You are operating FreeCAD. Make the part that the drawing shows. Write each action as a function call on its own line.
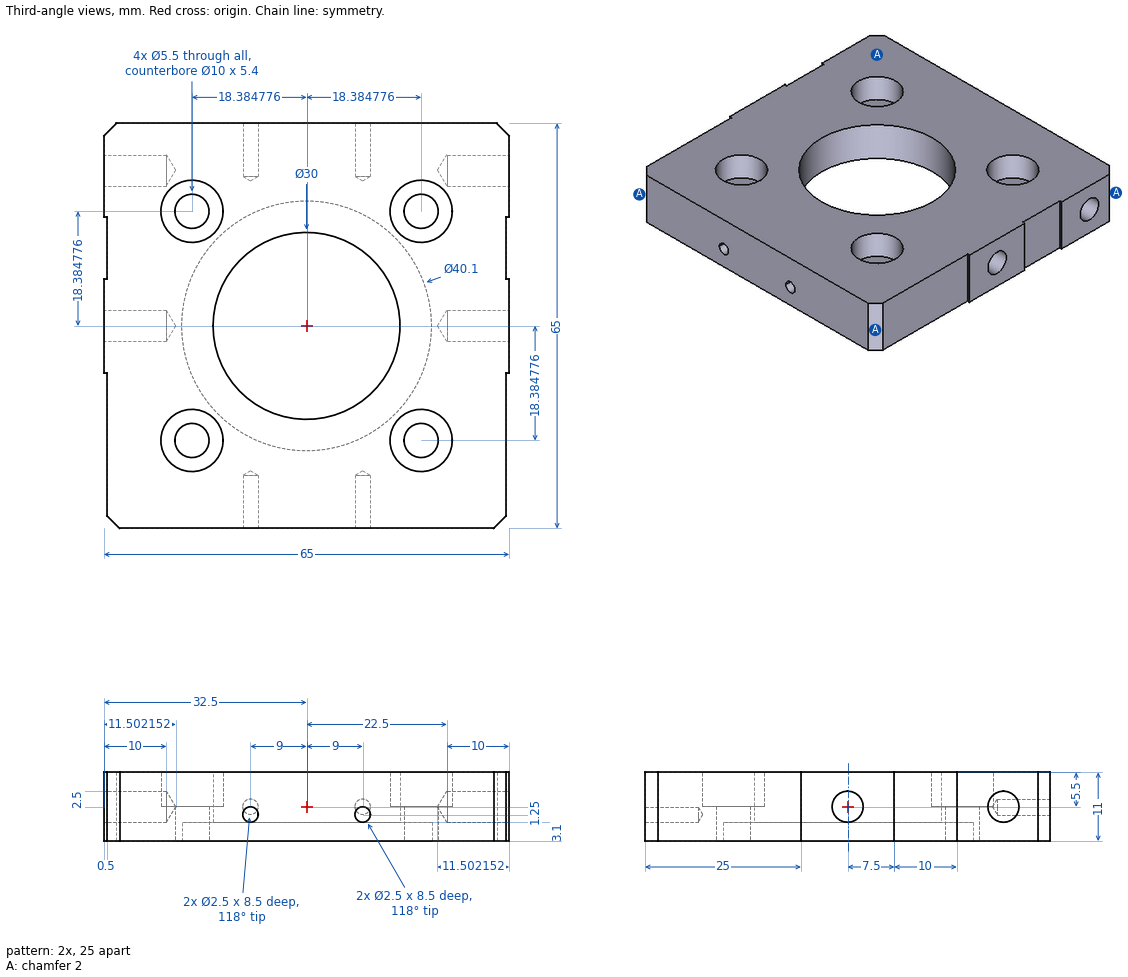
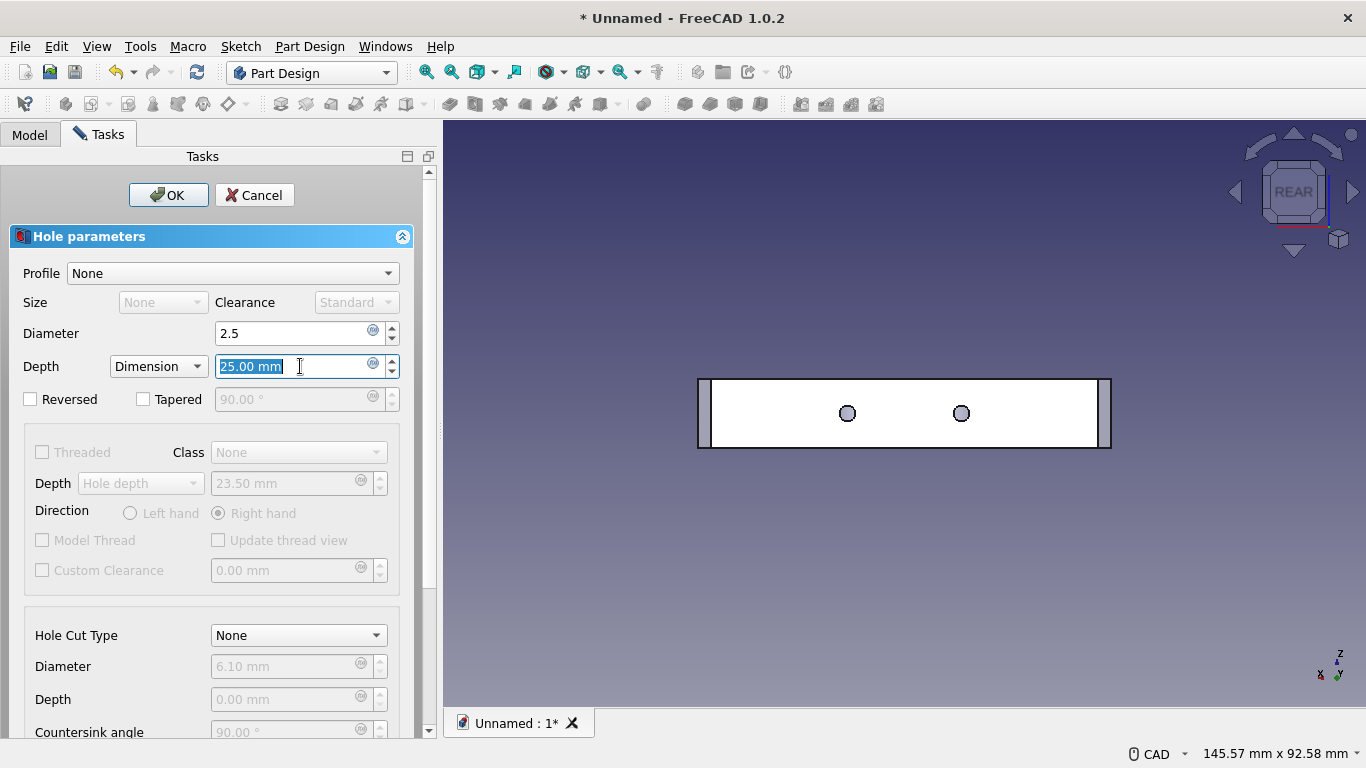
text(8.5)
key(Tab)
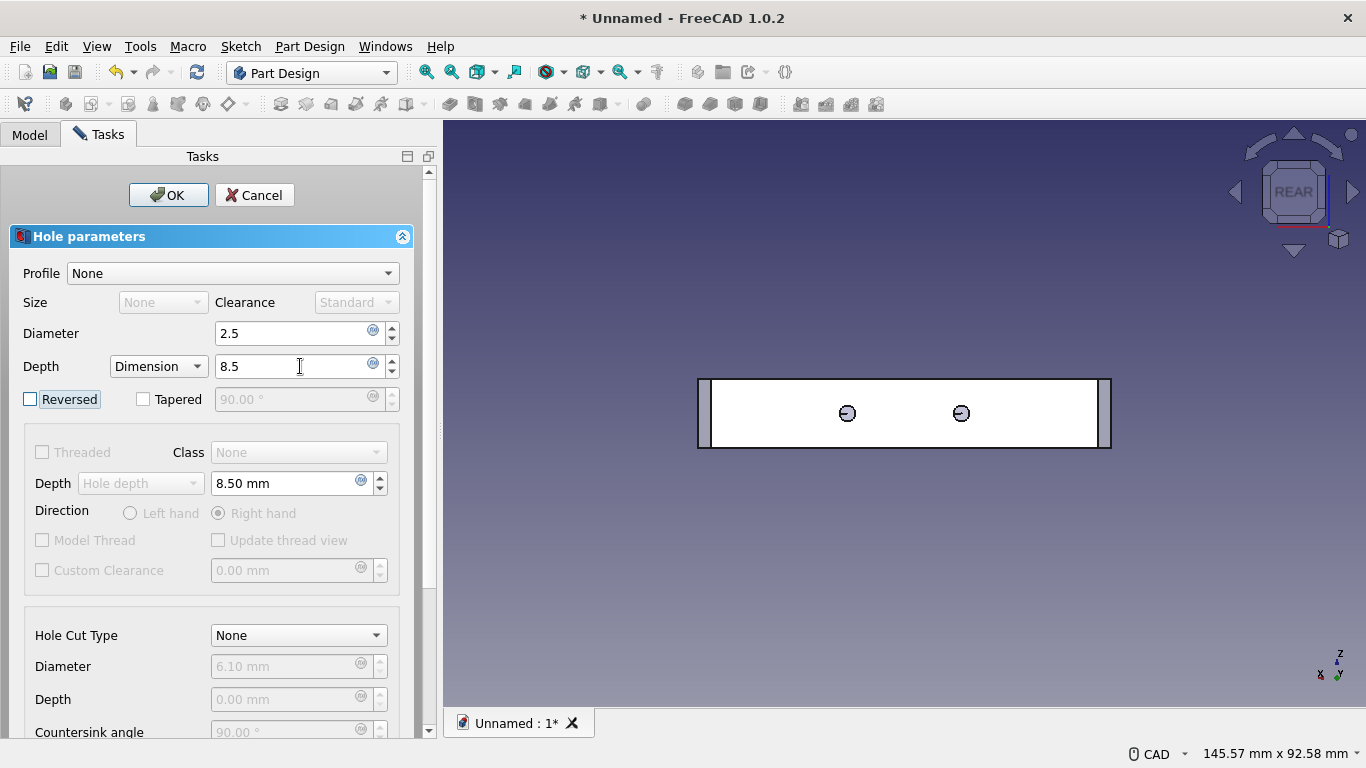
click(169, 195)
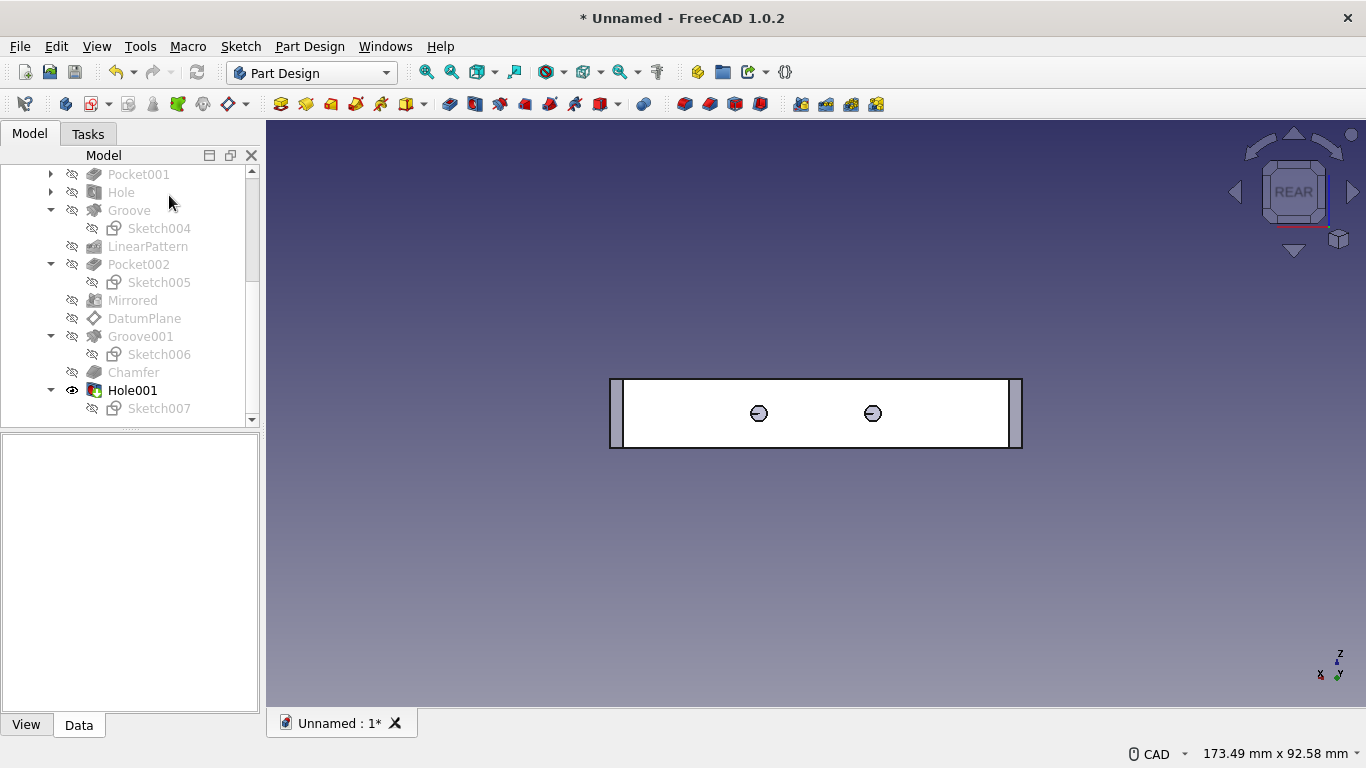
click(427, 72)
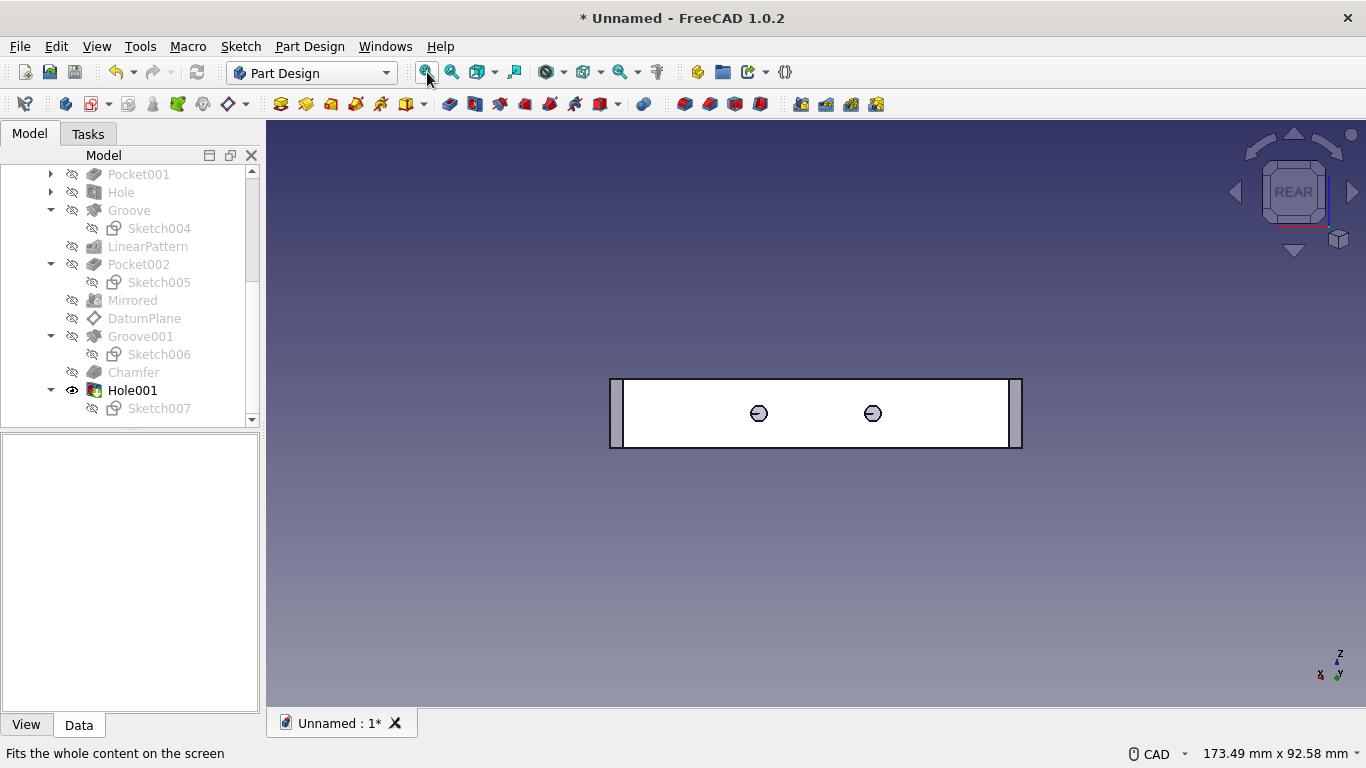
key(0)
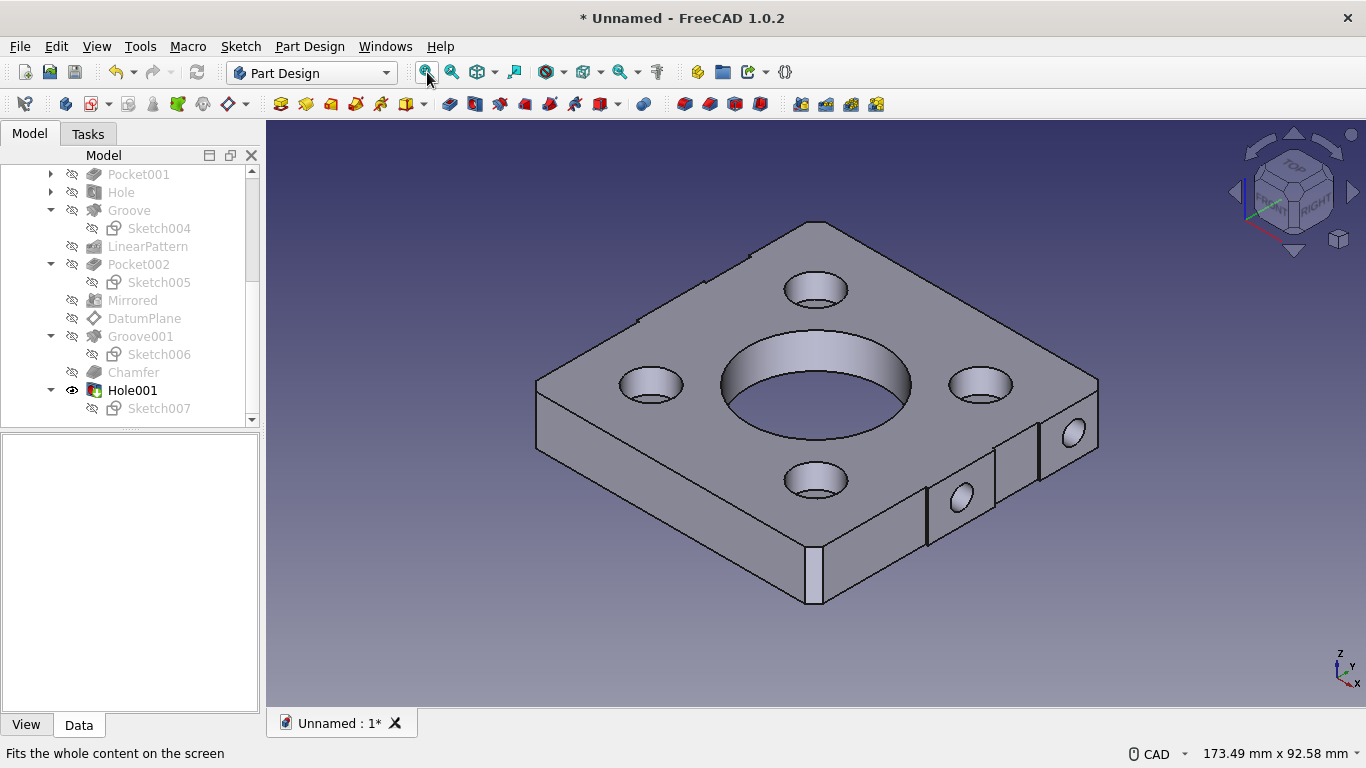
click(747, 541)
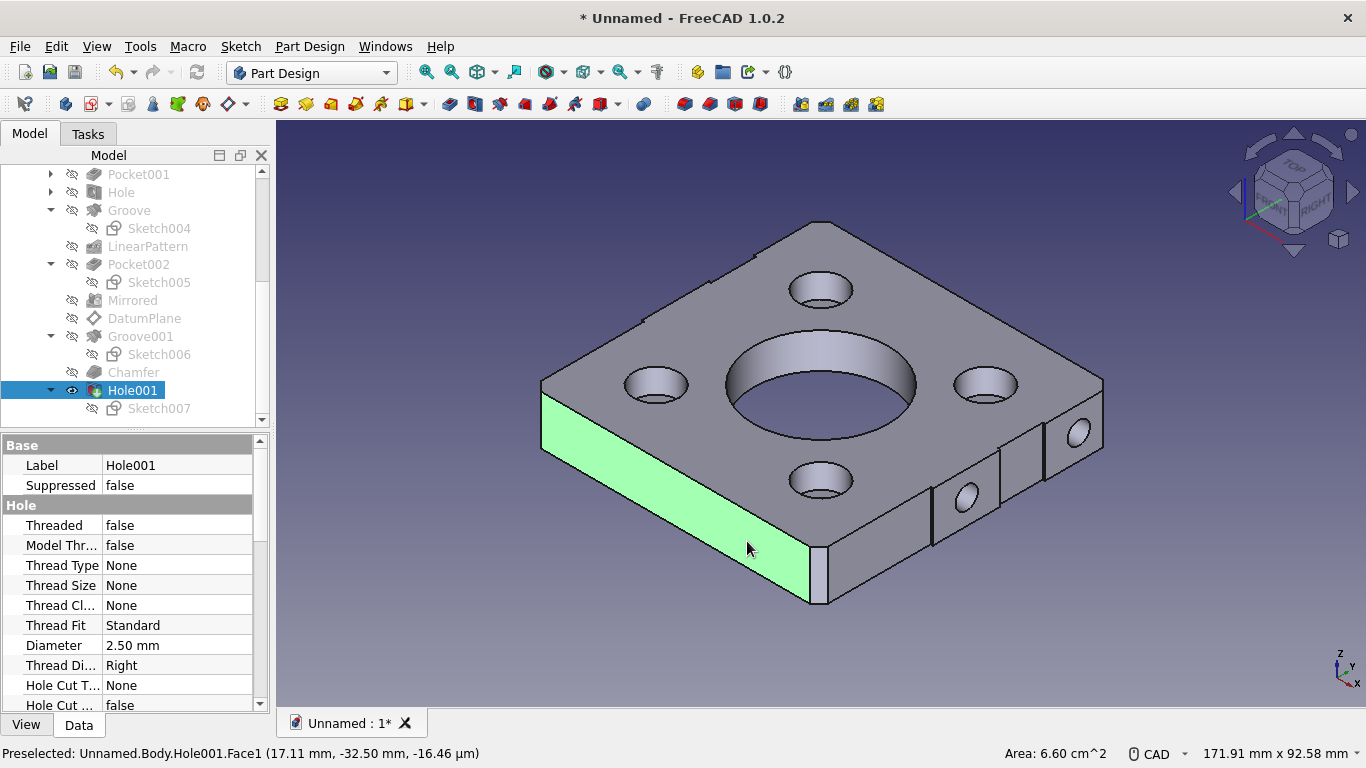
click(90, 104)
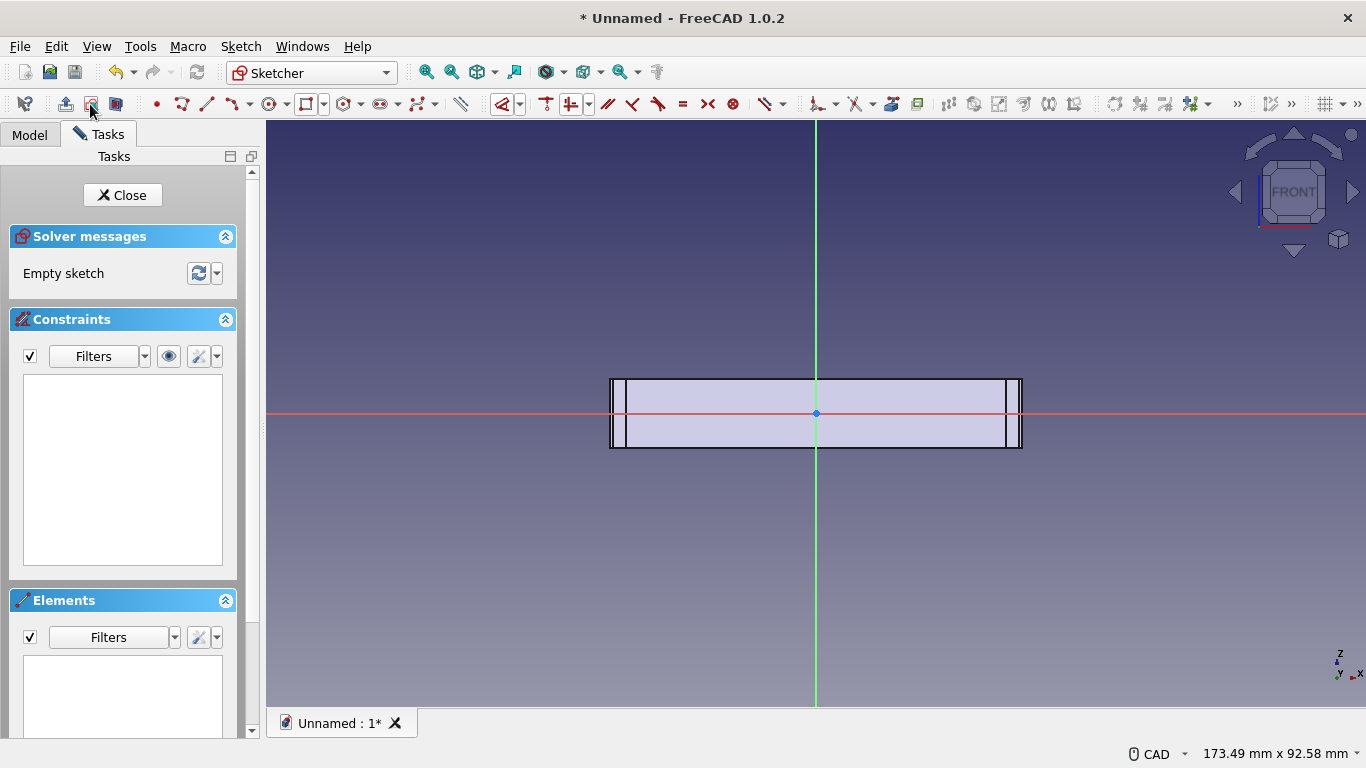
scroll(833, 423, up, 8)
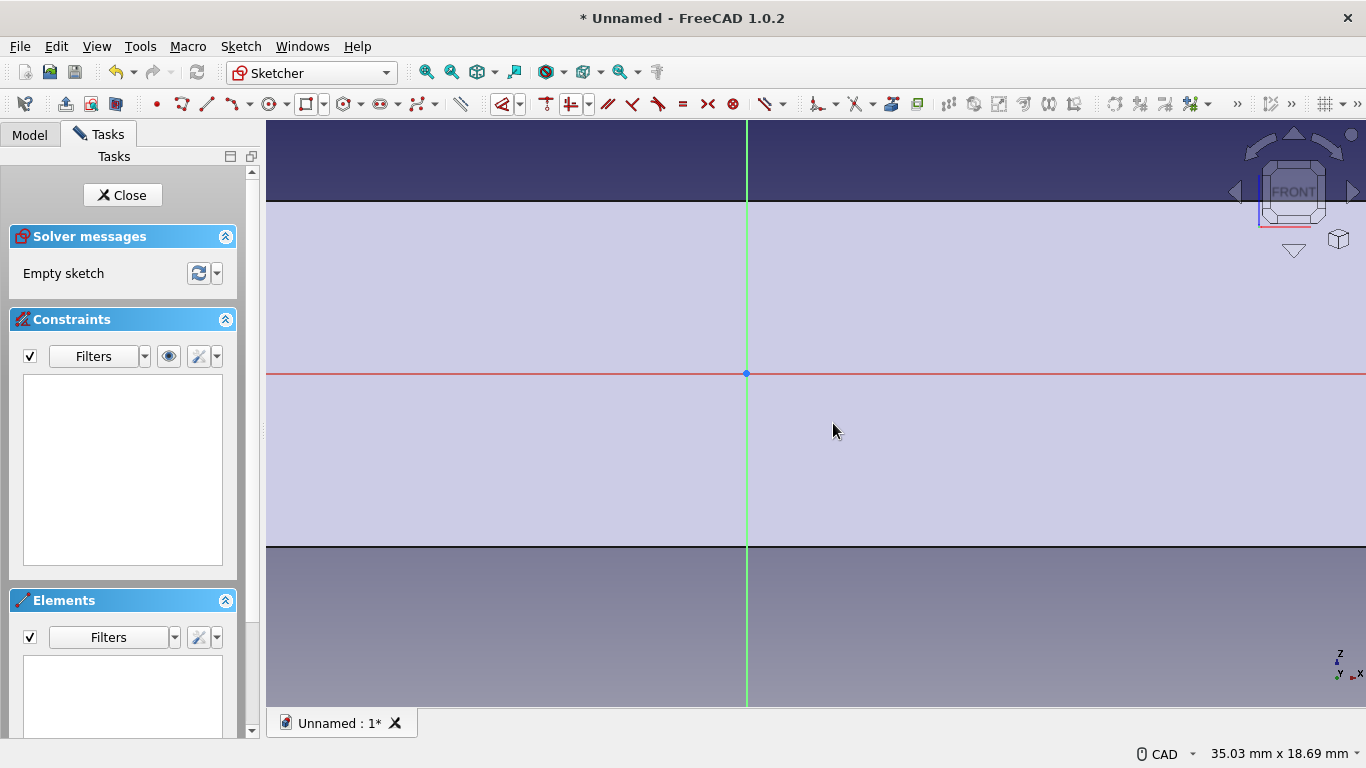
click(268, 104)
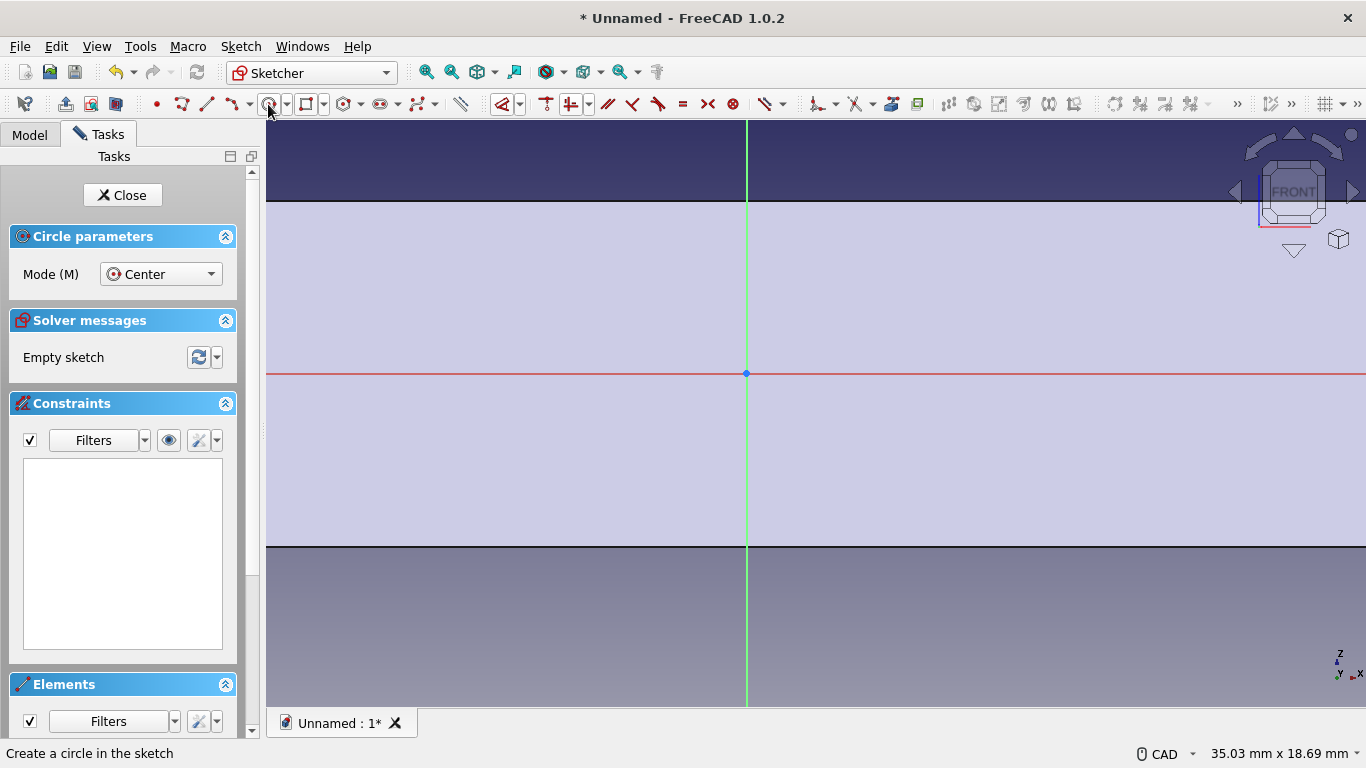
click(1029, 413)
click(1057, 441)